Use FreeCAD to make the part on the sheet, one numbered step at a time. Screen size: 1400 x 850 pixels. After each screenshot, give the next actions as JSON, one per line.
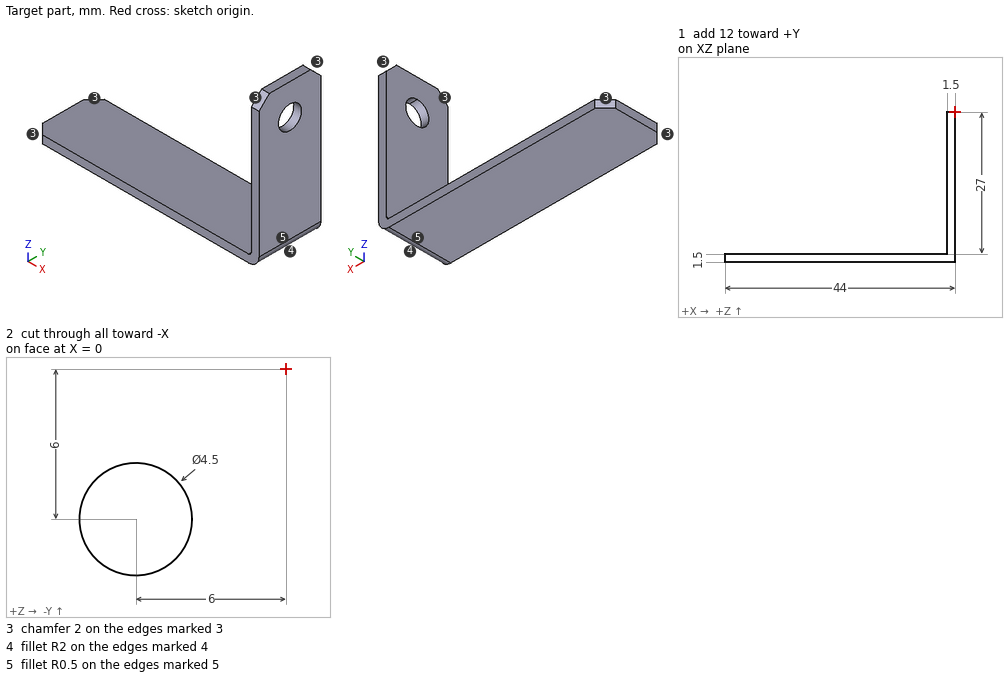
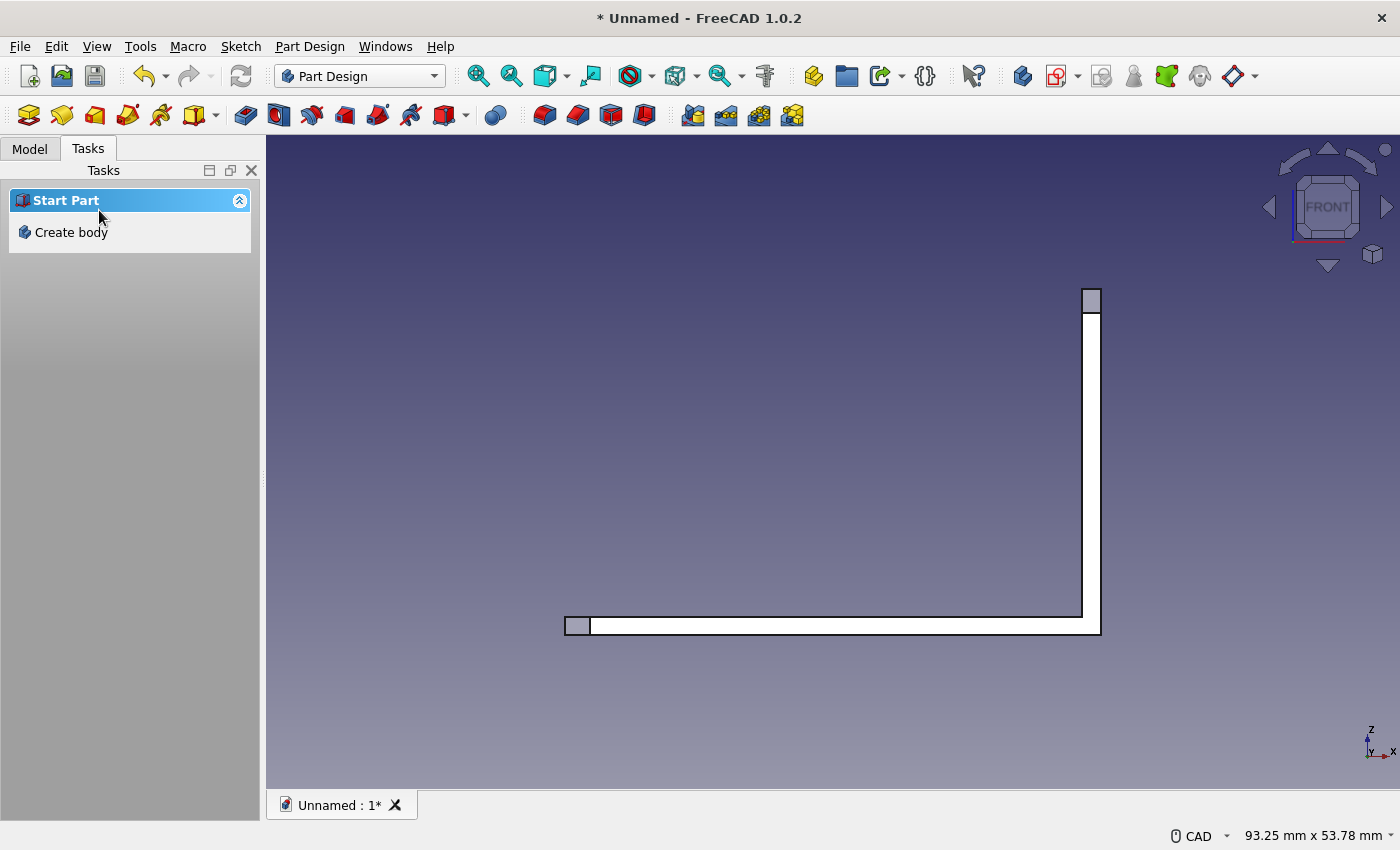
{"action": "key", "text": "3"}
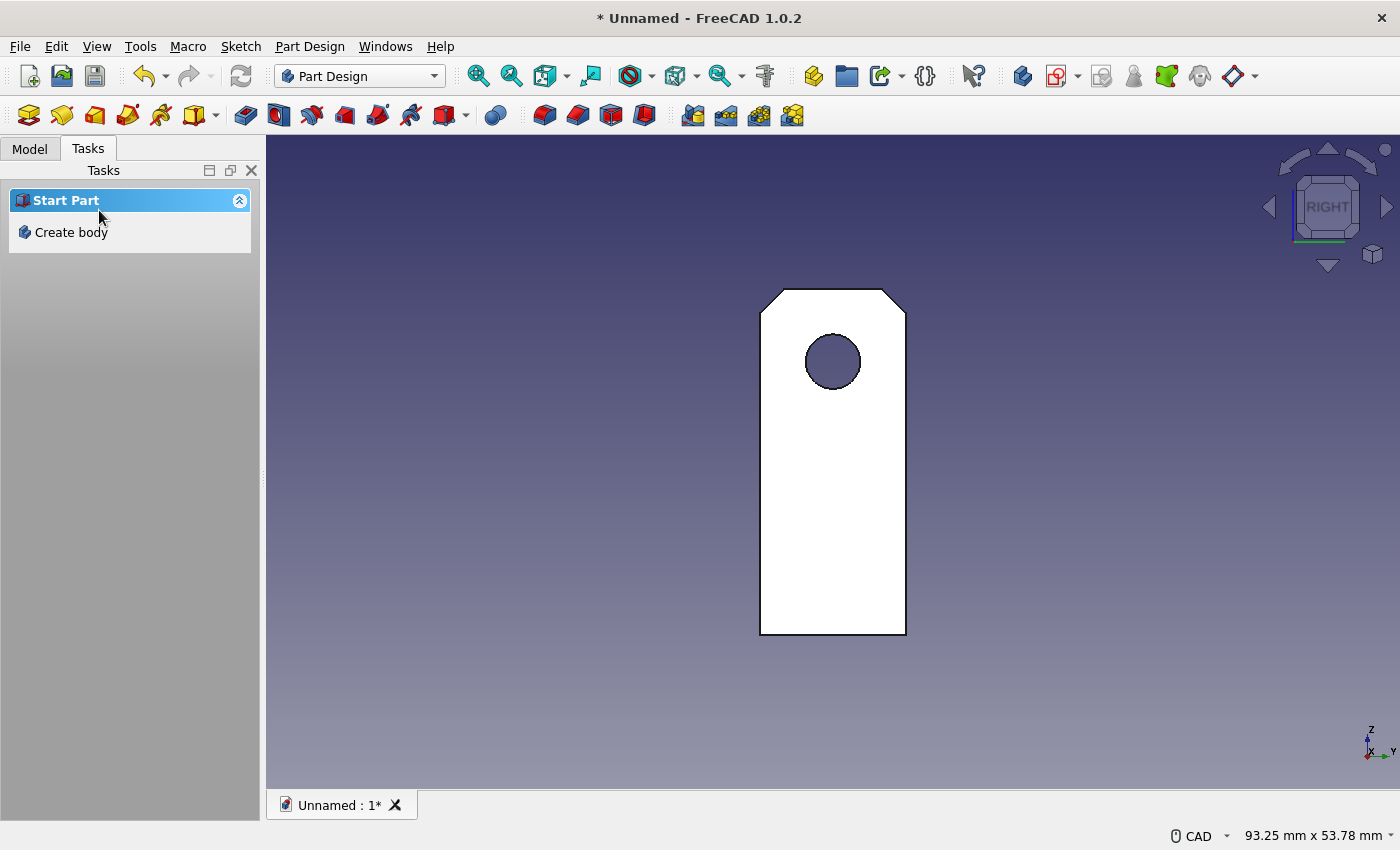
{"action": "left_click", "coordinate": [833, 634]}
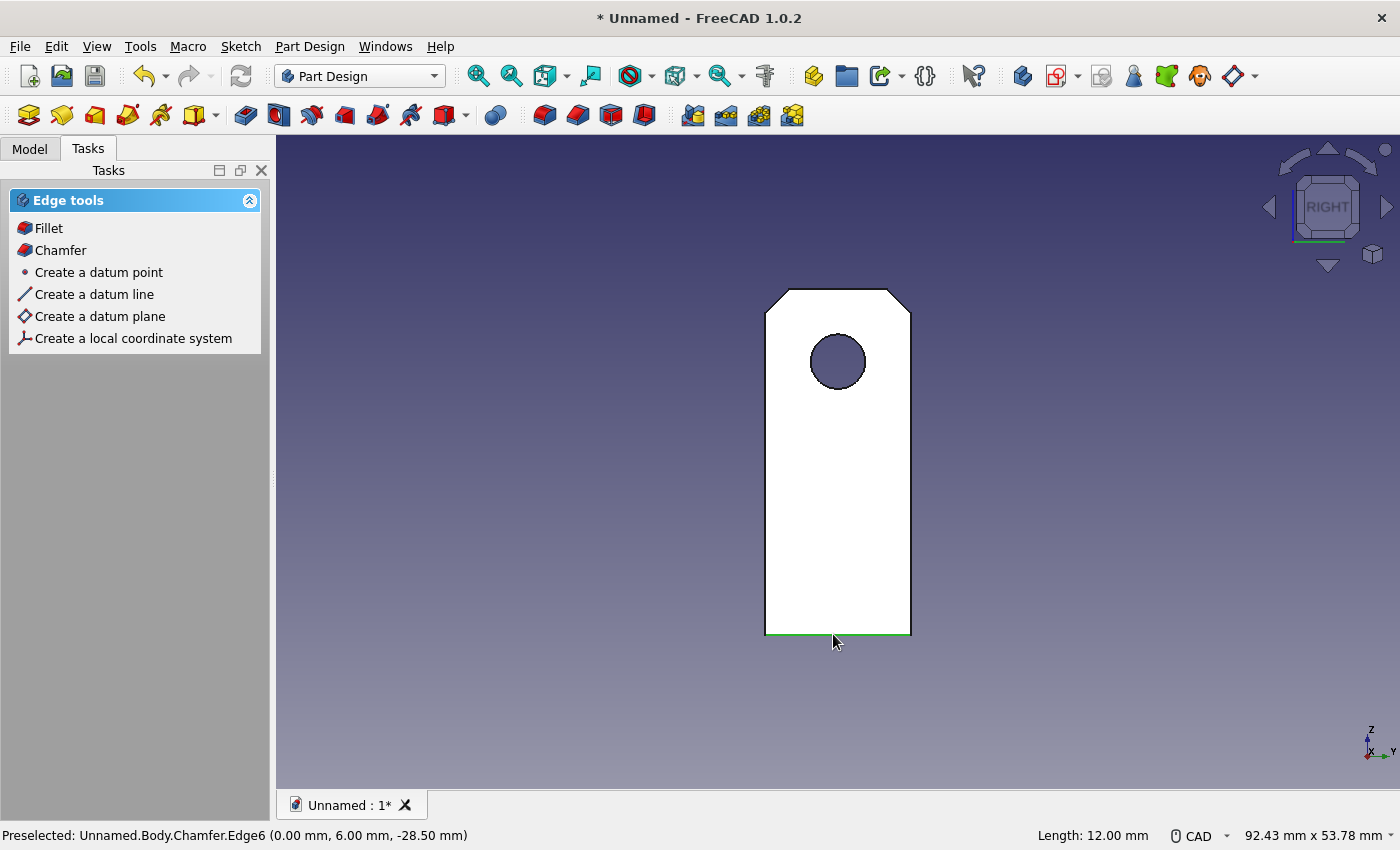
{"action": "left_click", "coordinate": [545, 116]}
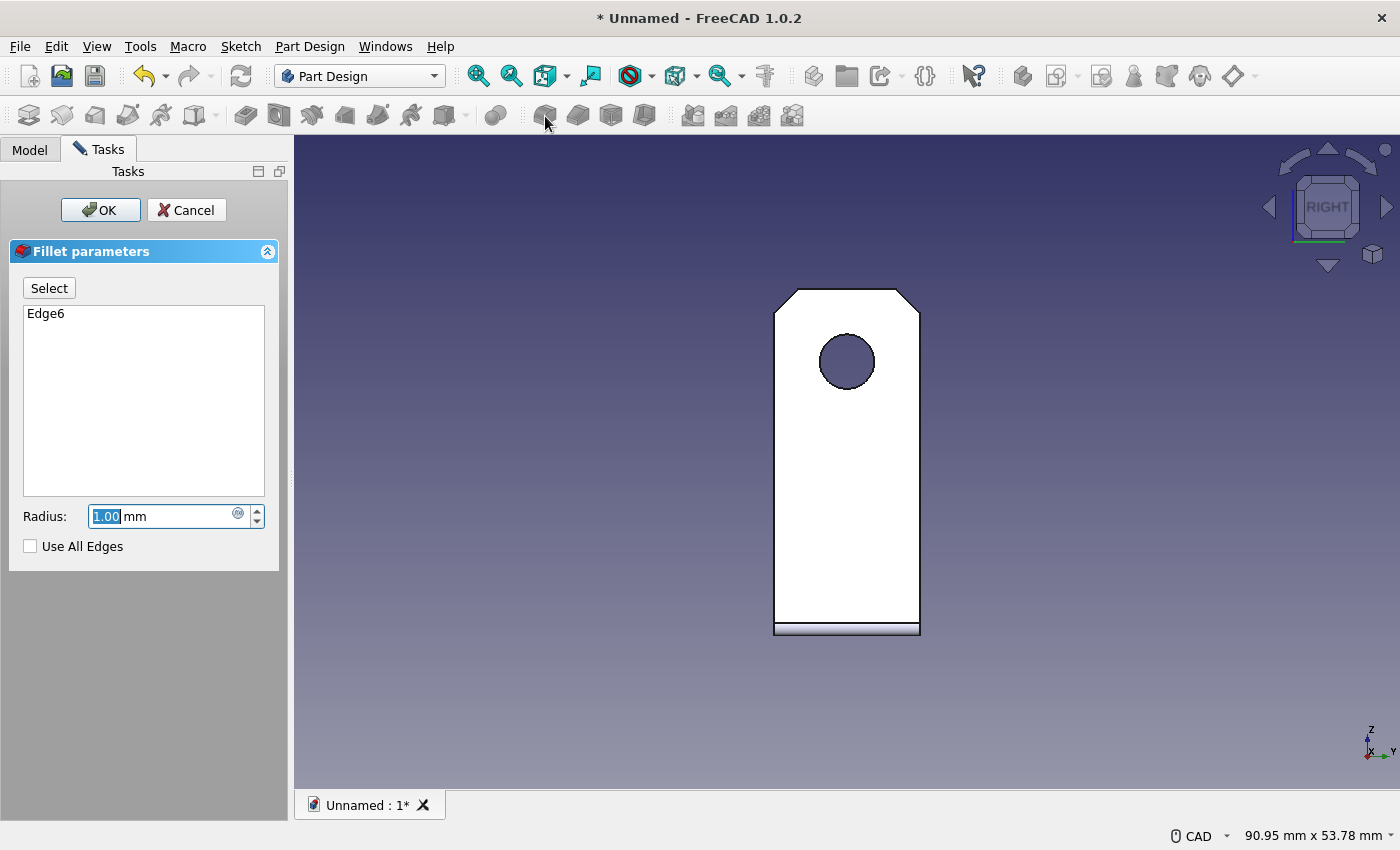
{"action": "type", "text": "2"}
{"action": "key", "text": "Tab"}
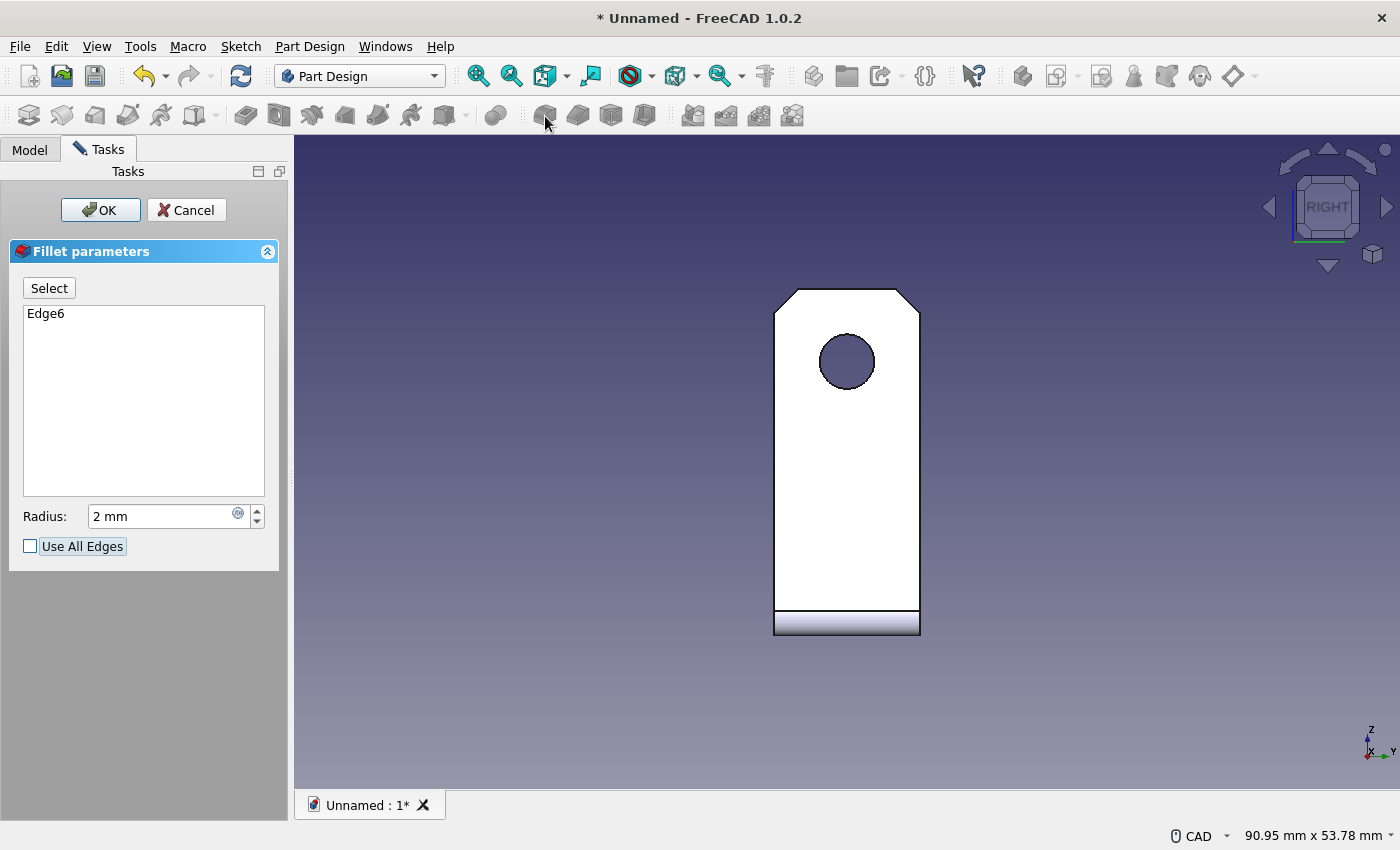
{"action": "left_click", "coordinate": [101, 210]}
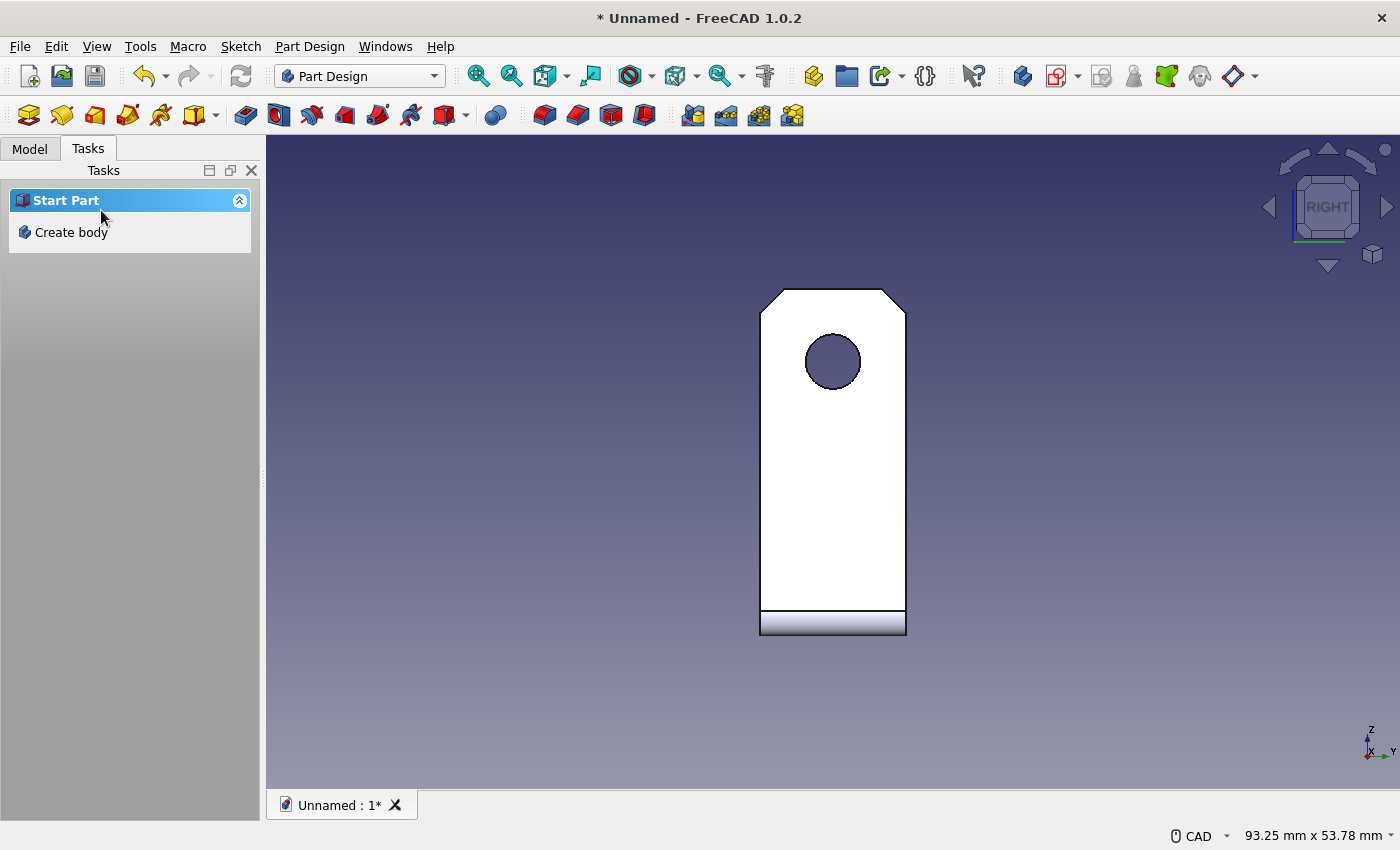
{"action": "key", "text": "0"}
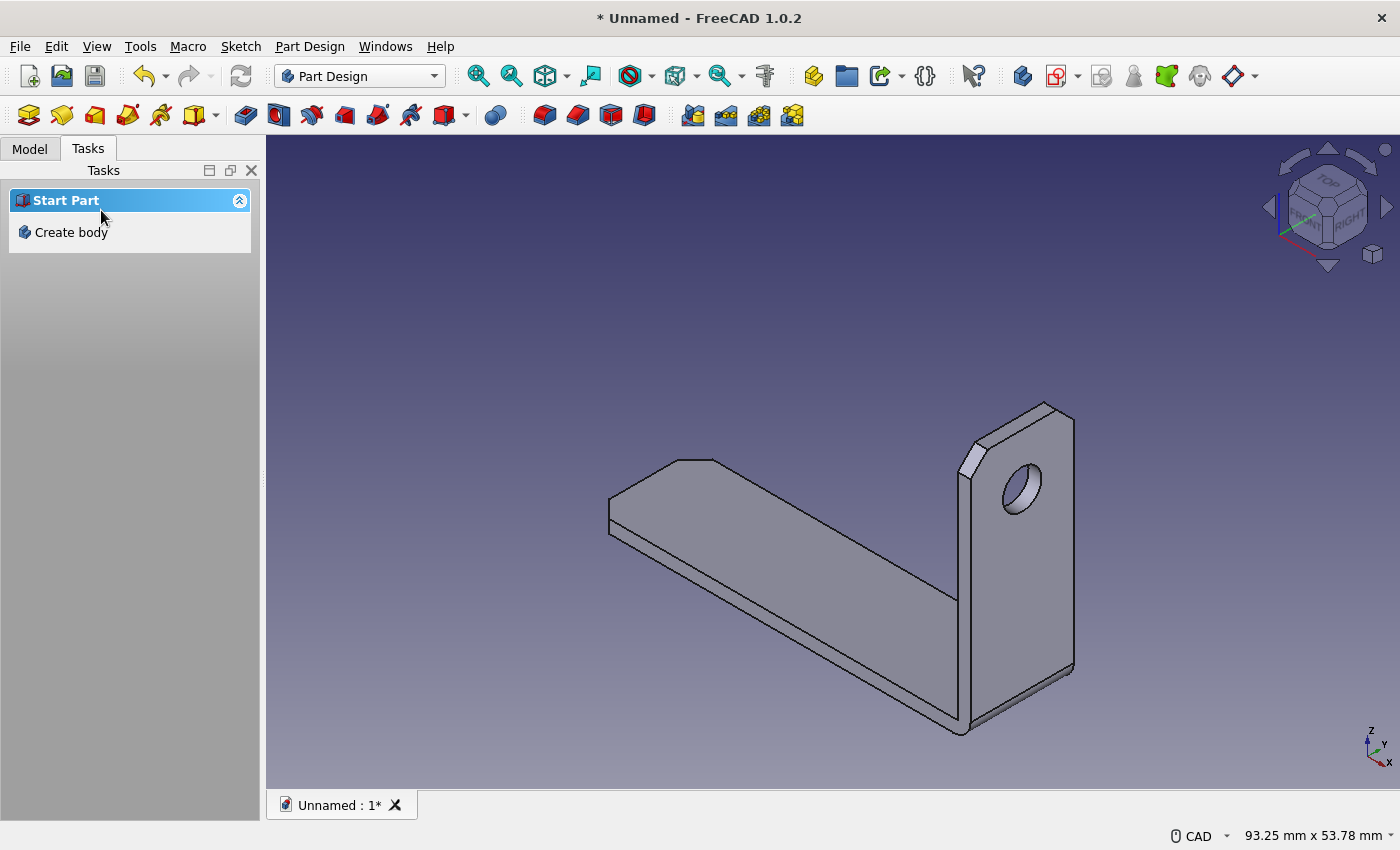
{"action": "key", "text": "2"}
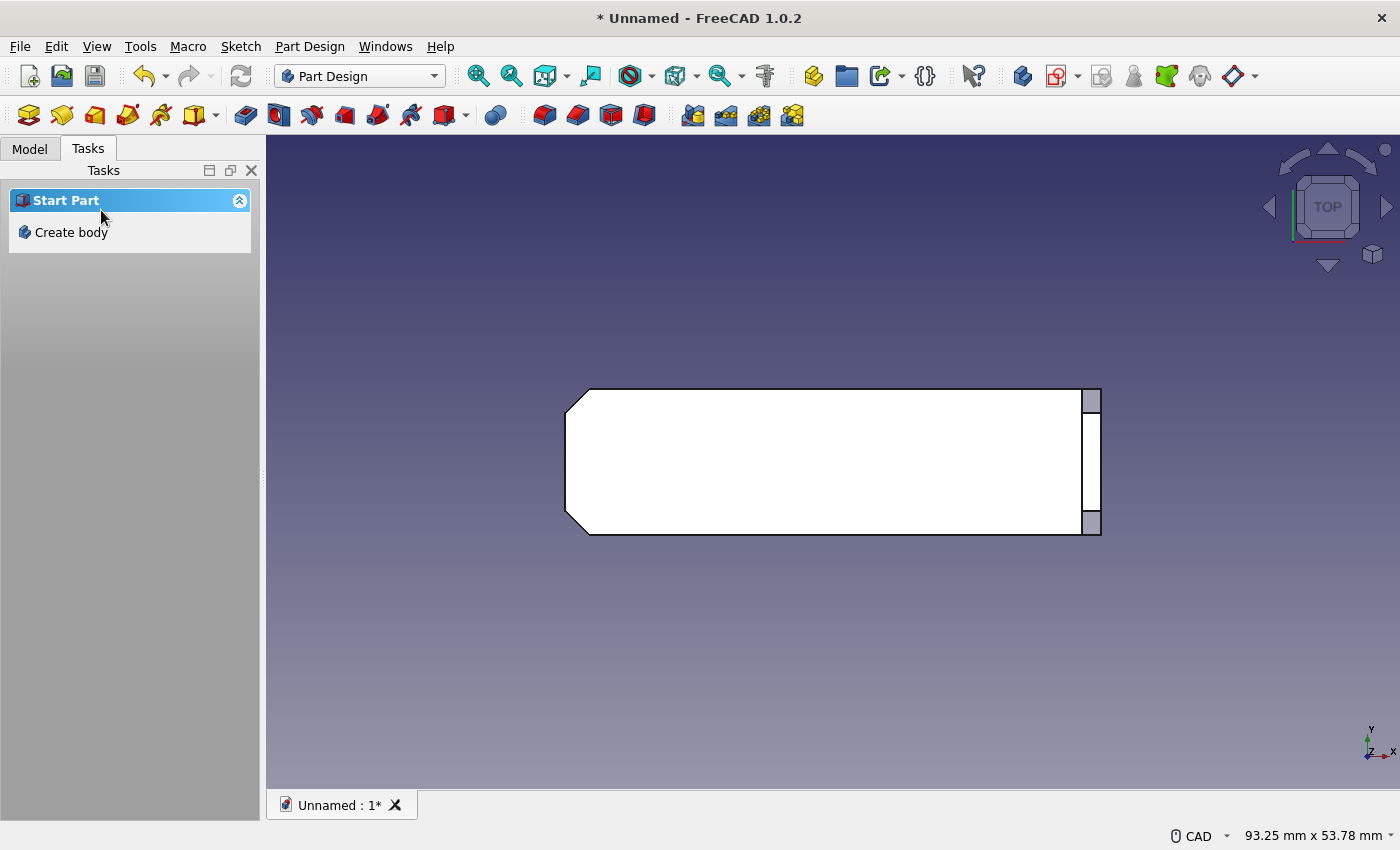
{"action": "key", "text": "1"}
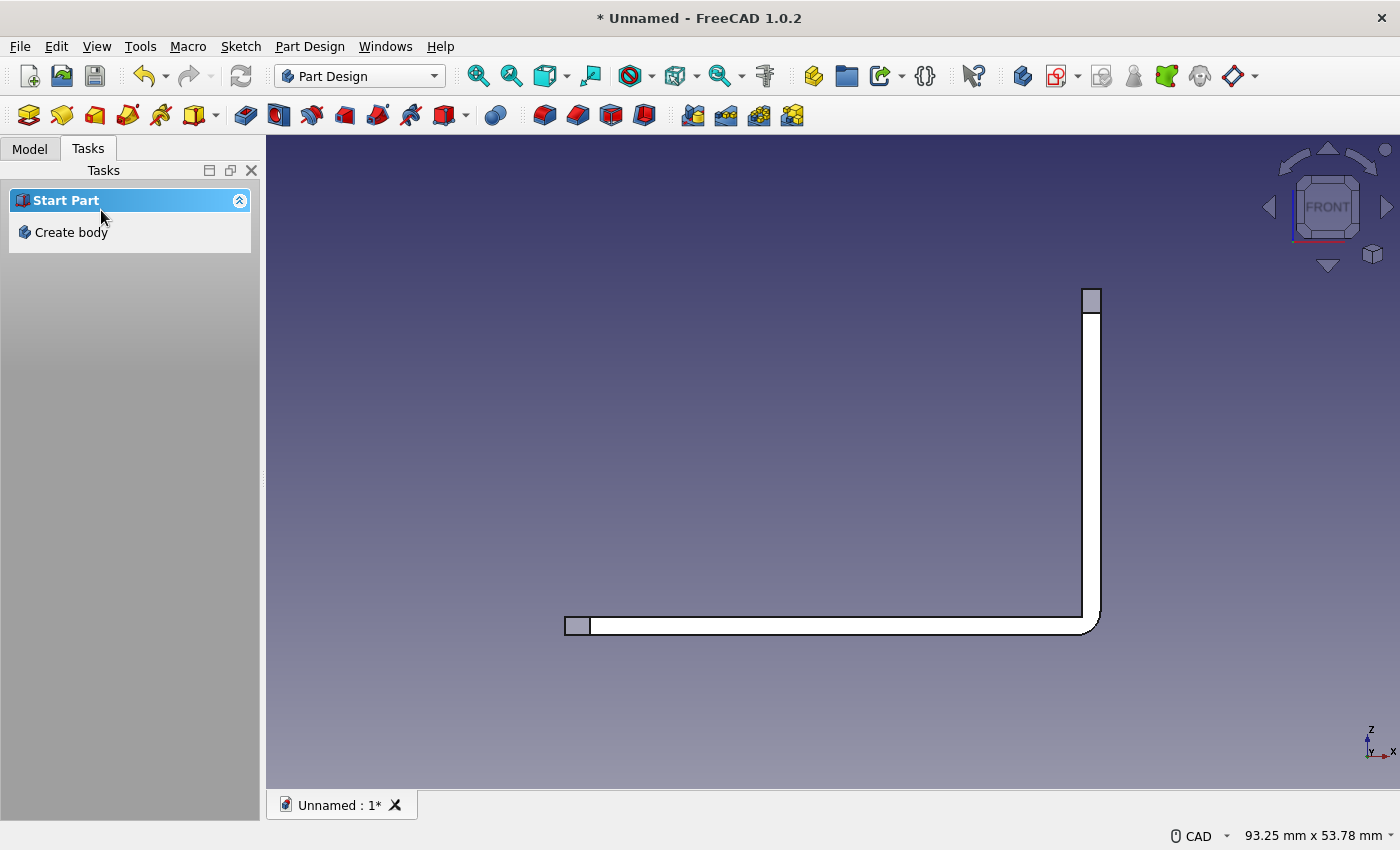
{"action": "key", "text": "3"}